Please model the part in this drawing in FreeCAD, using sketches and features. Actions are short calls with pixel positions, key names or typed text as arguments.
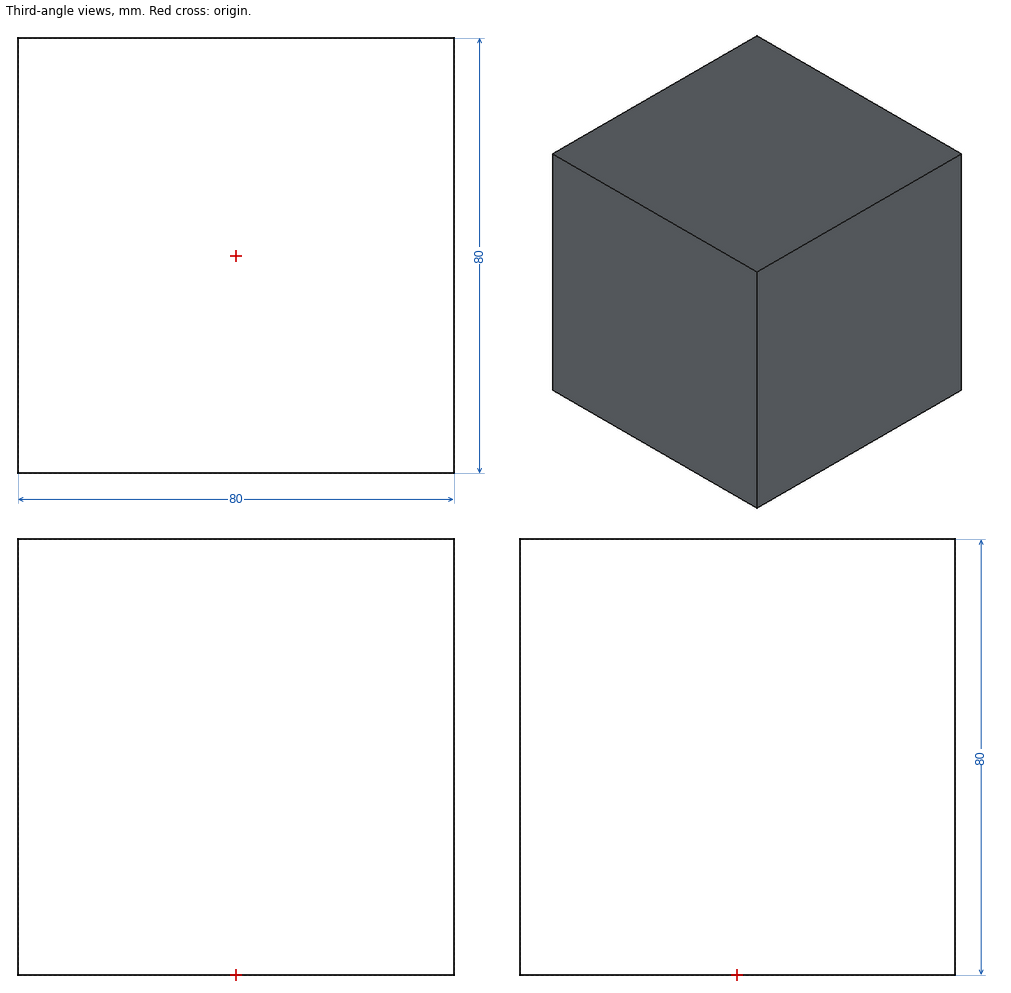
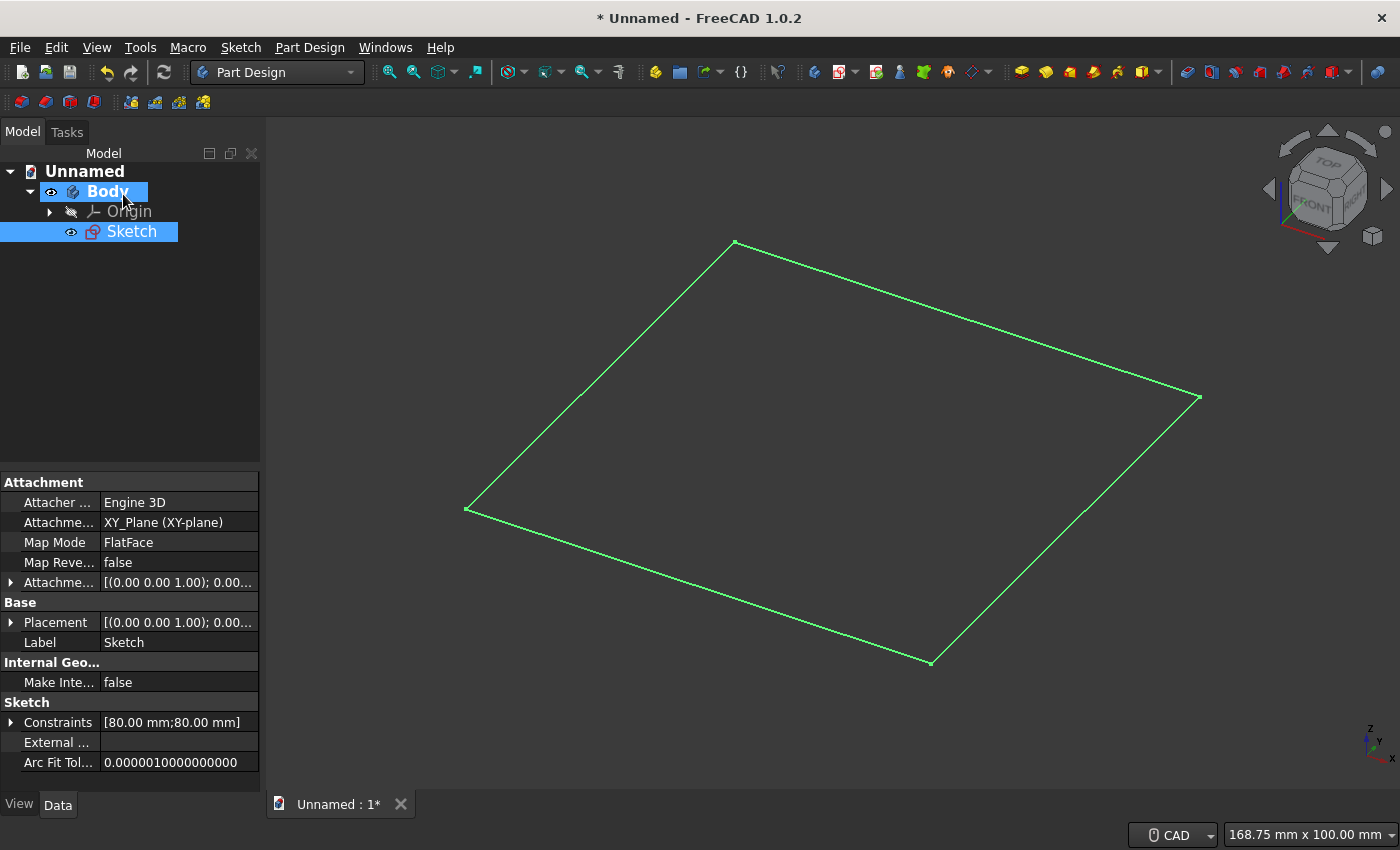
click(1022, 72)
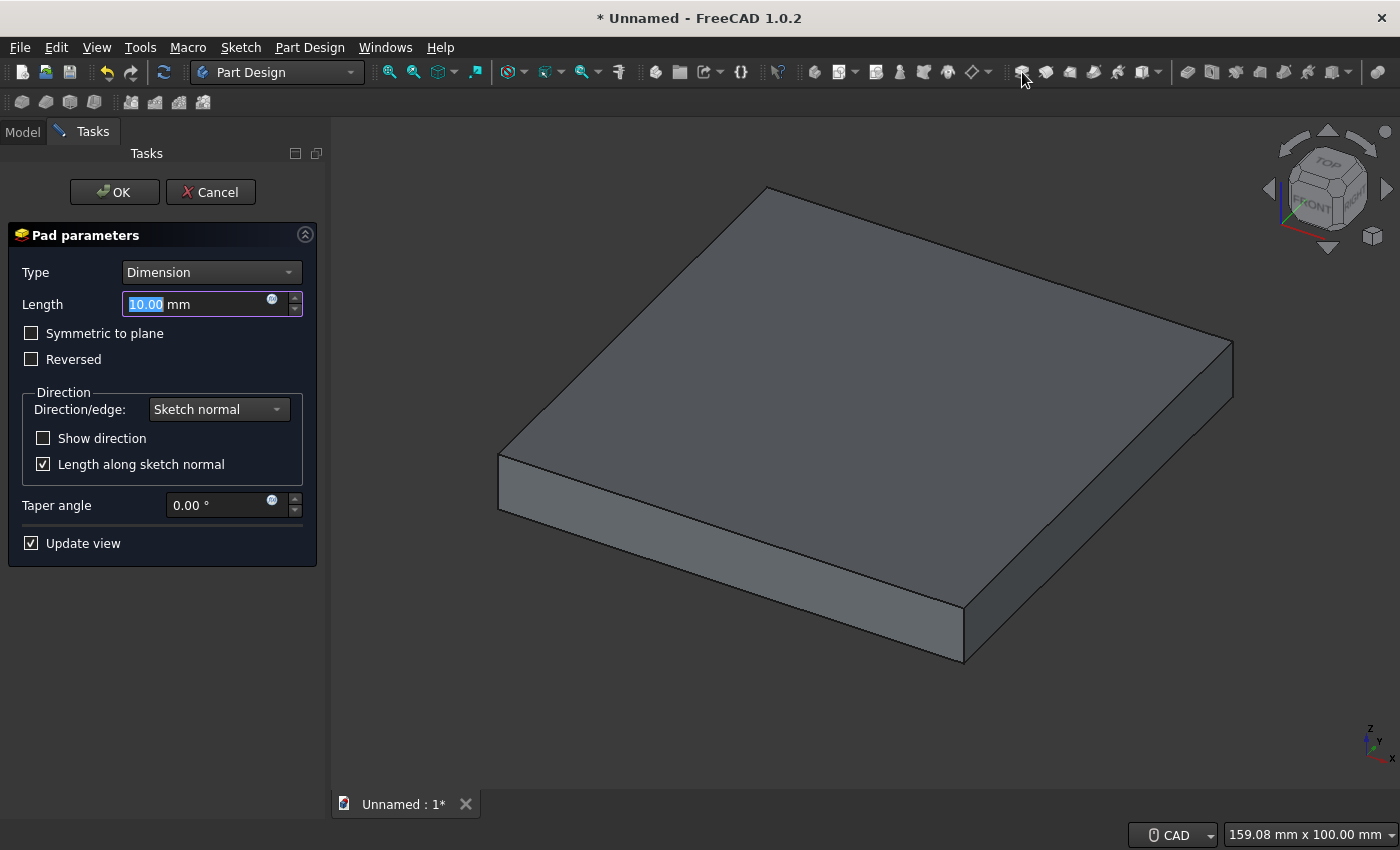
text(80)
key(Tab)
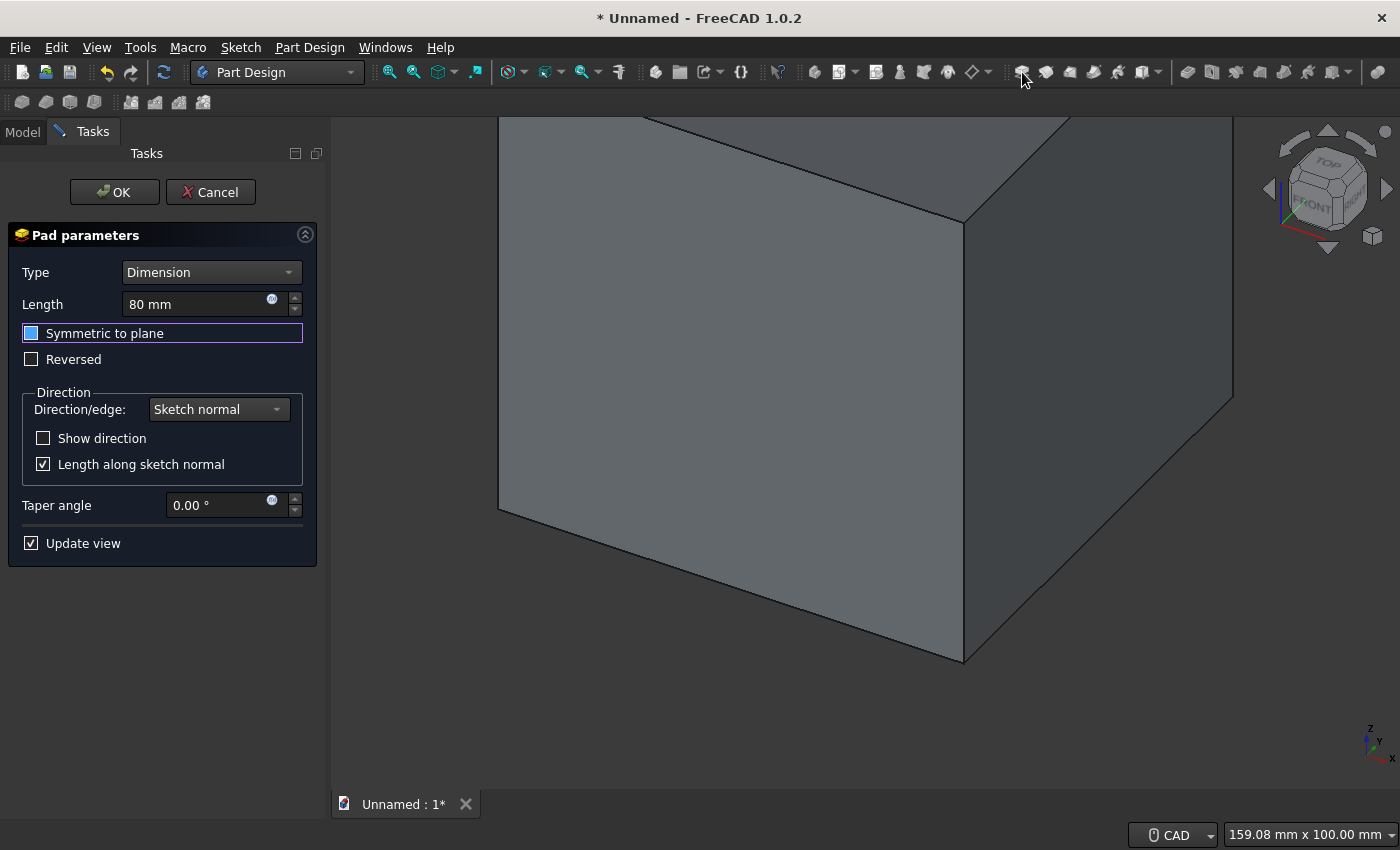
click(115, 192)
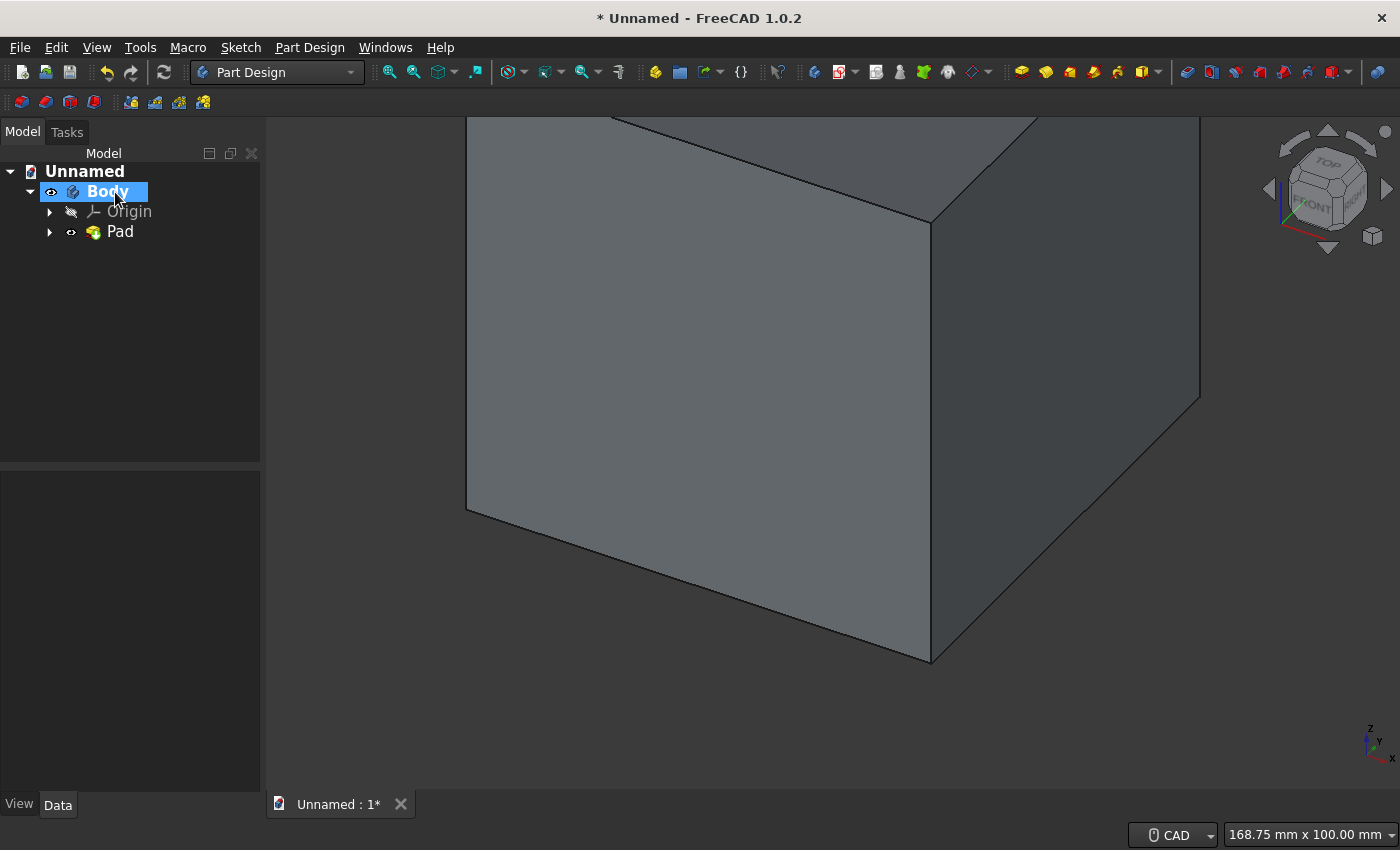
key(0)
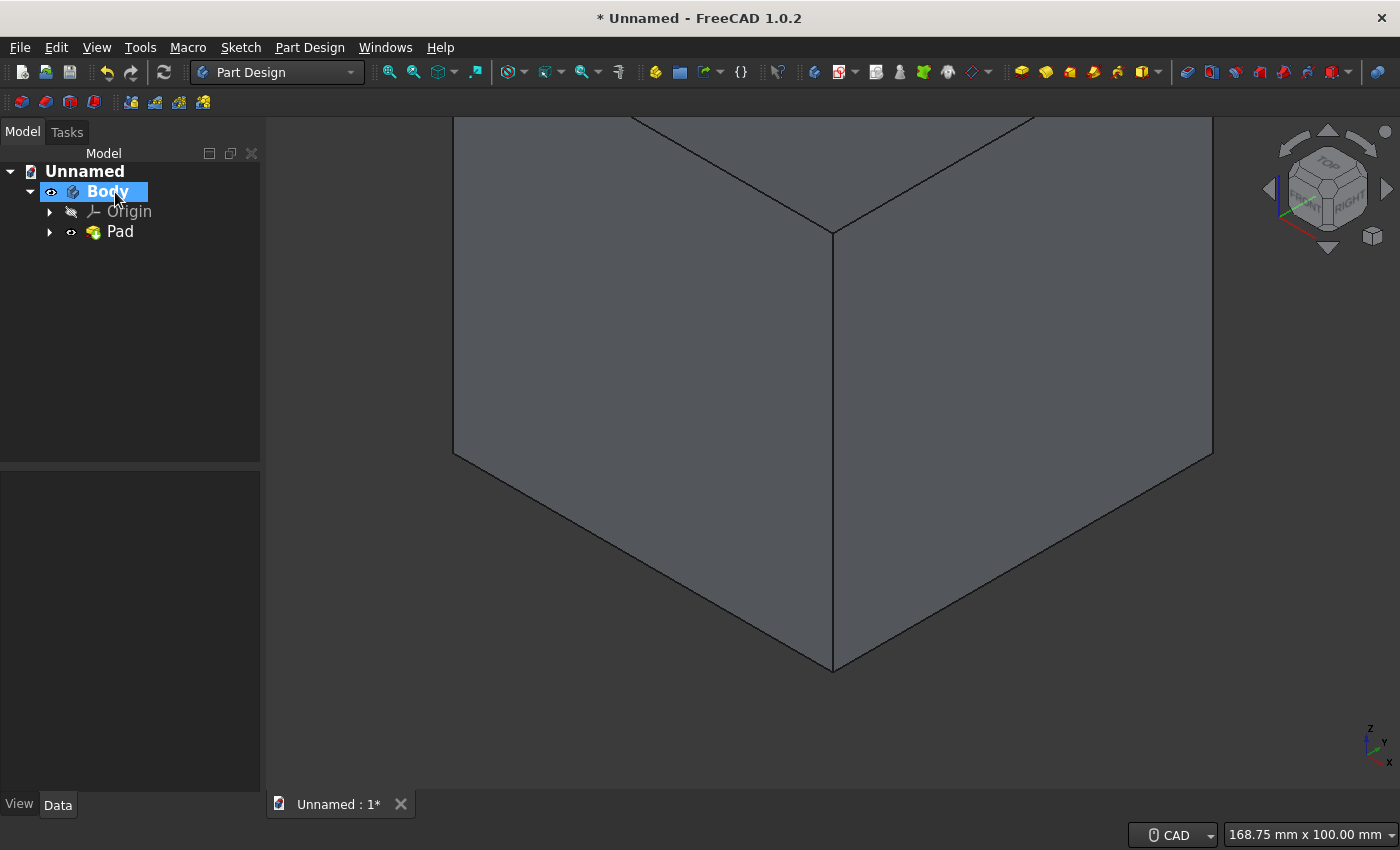
click(390, 72)